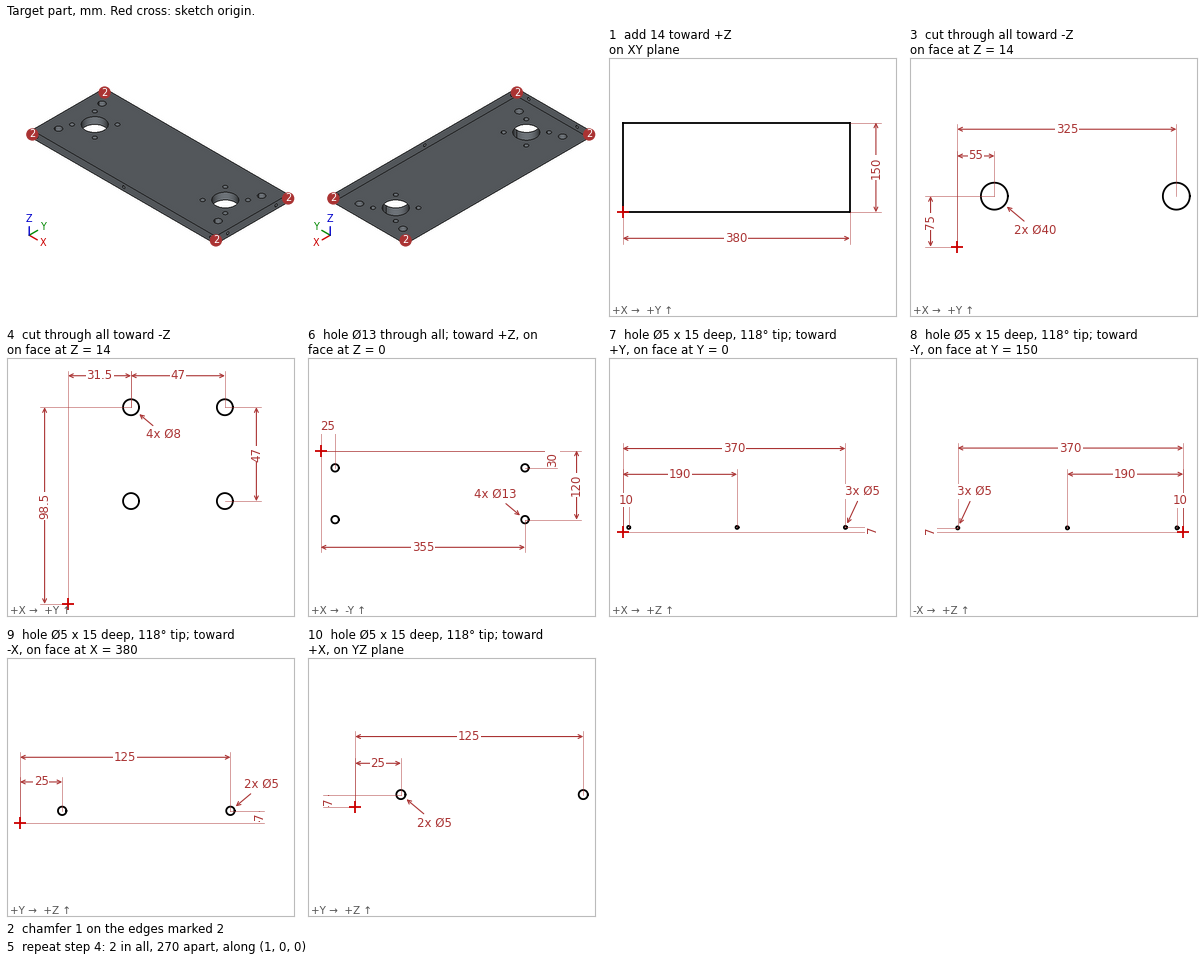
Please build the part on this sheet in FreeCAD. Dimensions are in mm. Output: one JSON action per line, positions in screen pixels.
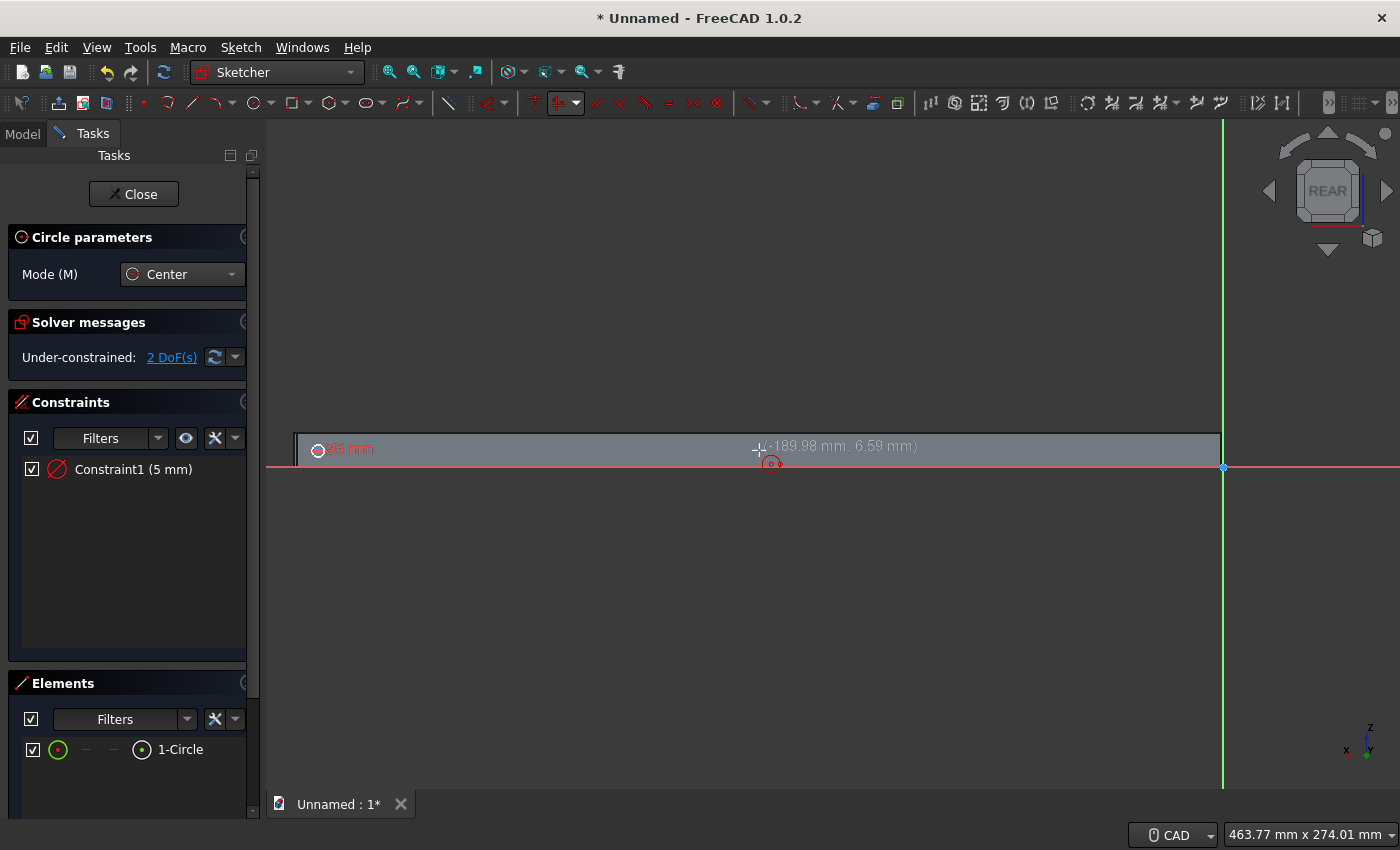
{"action": "left_click", "coordinate": [759, 450]}
{"action": "mouse_move", "coordinate": [763, 446]}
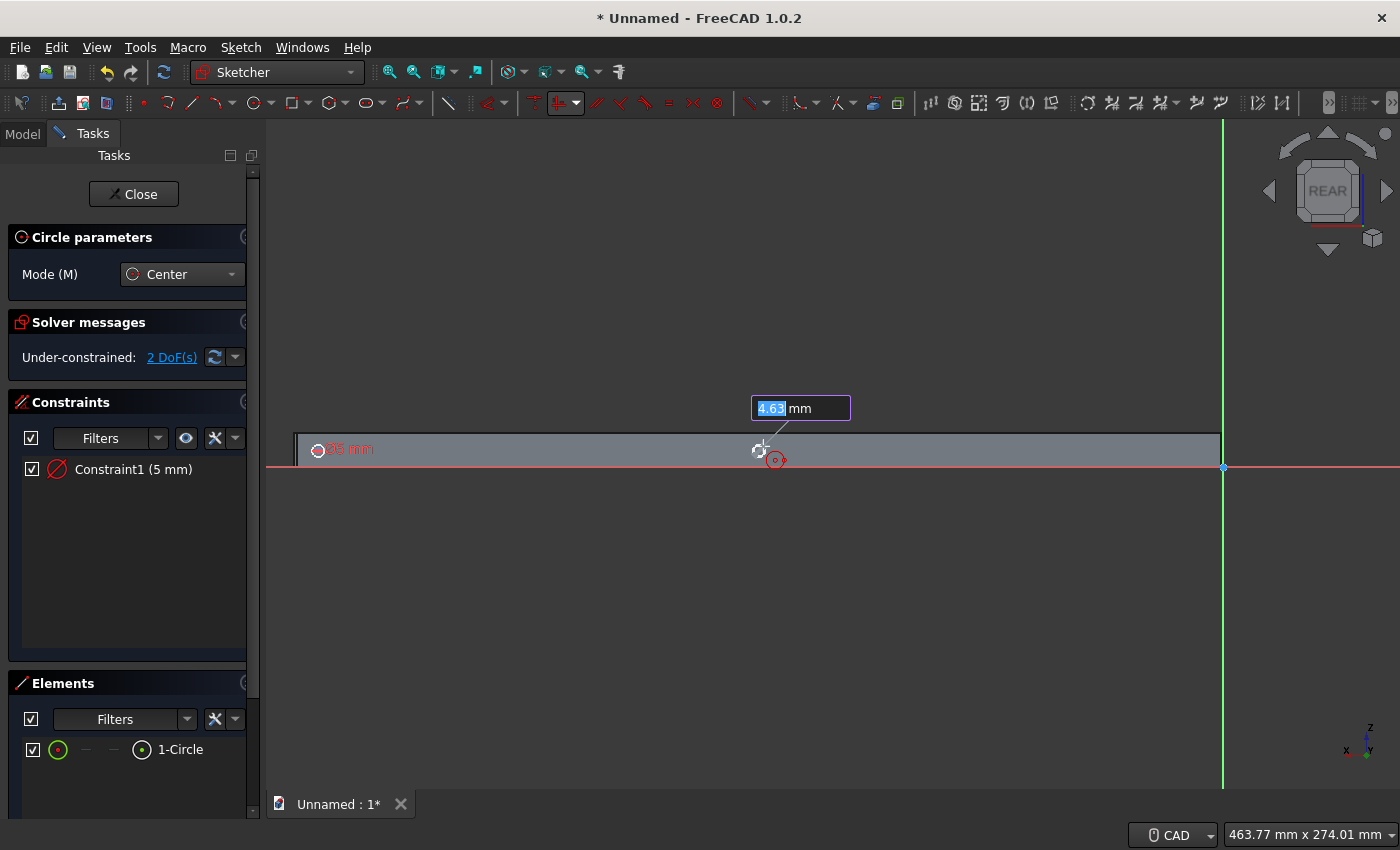
{"action": "type", "text": "5"}
{"action": "key", "text": "Return"}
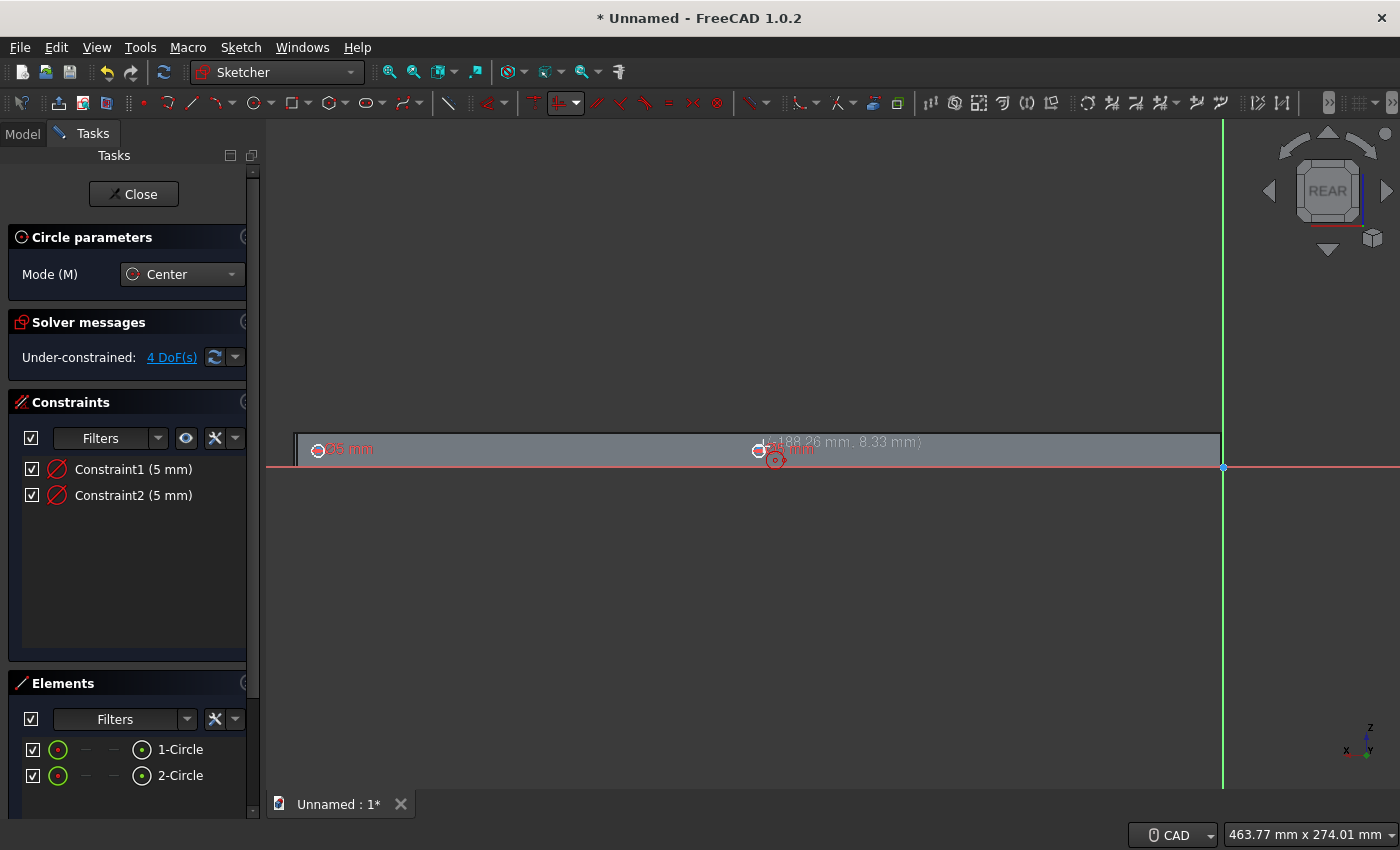
{"action": "scroll", "coordinate": [1199, 450], "scroll_direction": "up", "scroll_amount": 7}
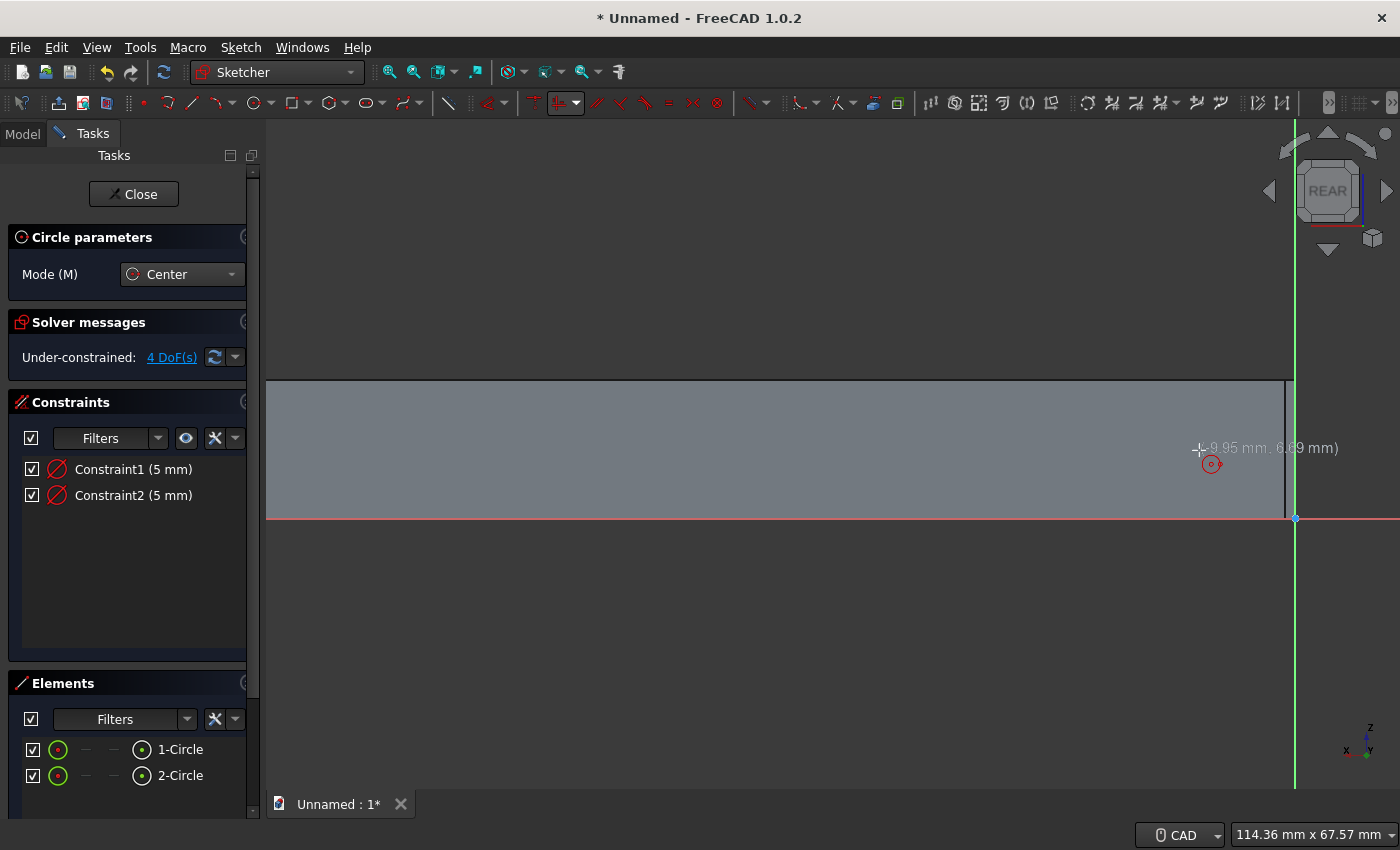
{"action": "scroll", "coordinate": [1025, 450], "scroll_direction": "down", "scroll_amount": 9}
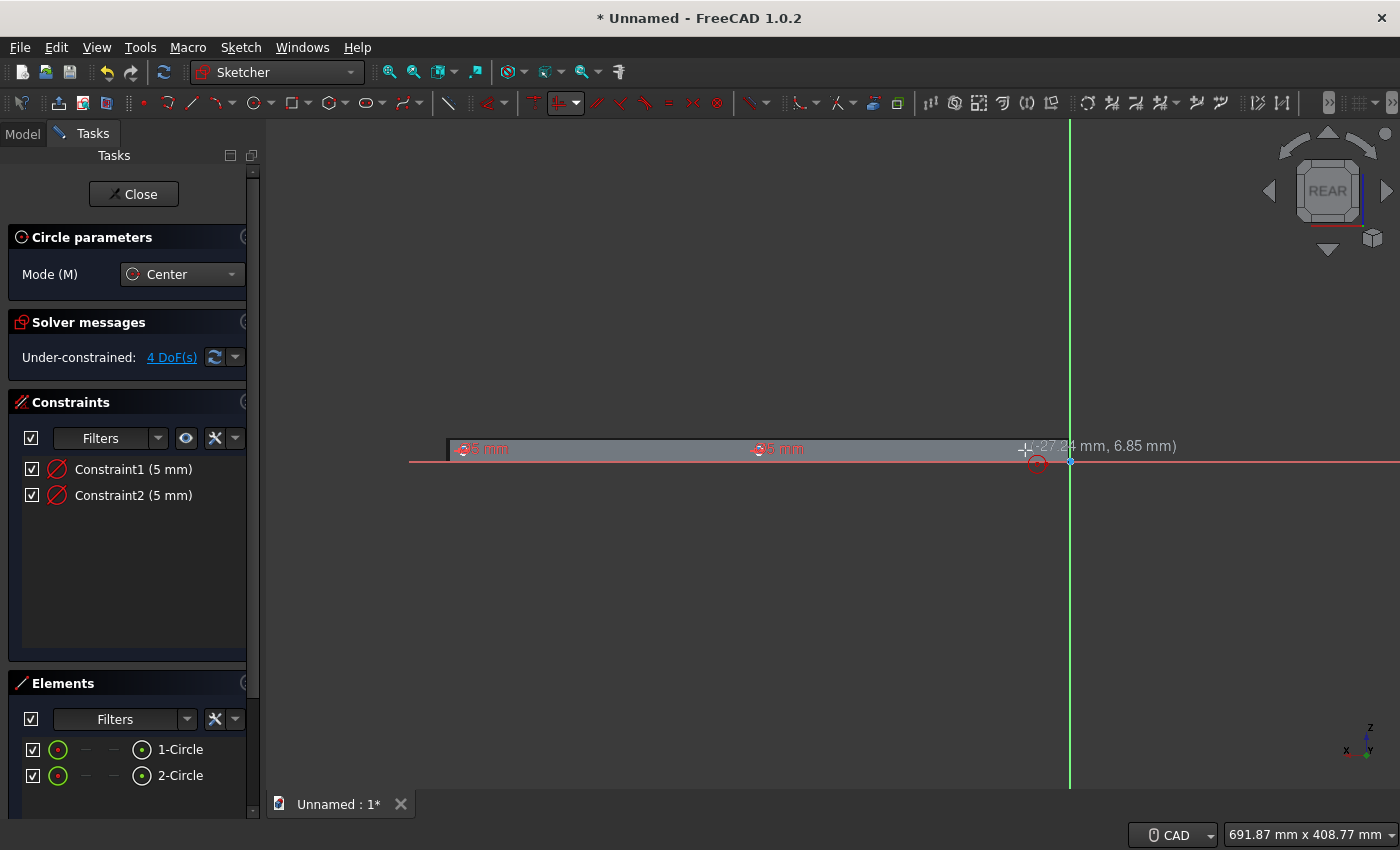
{"action": "scroll", "coordinate": [1054, 450], "scroll_direction": "up", "scroll_amount": 2}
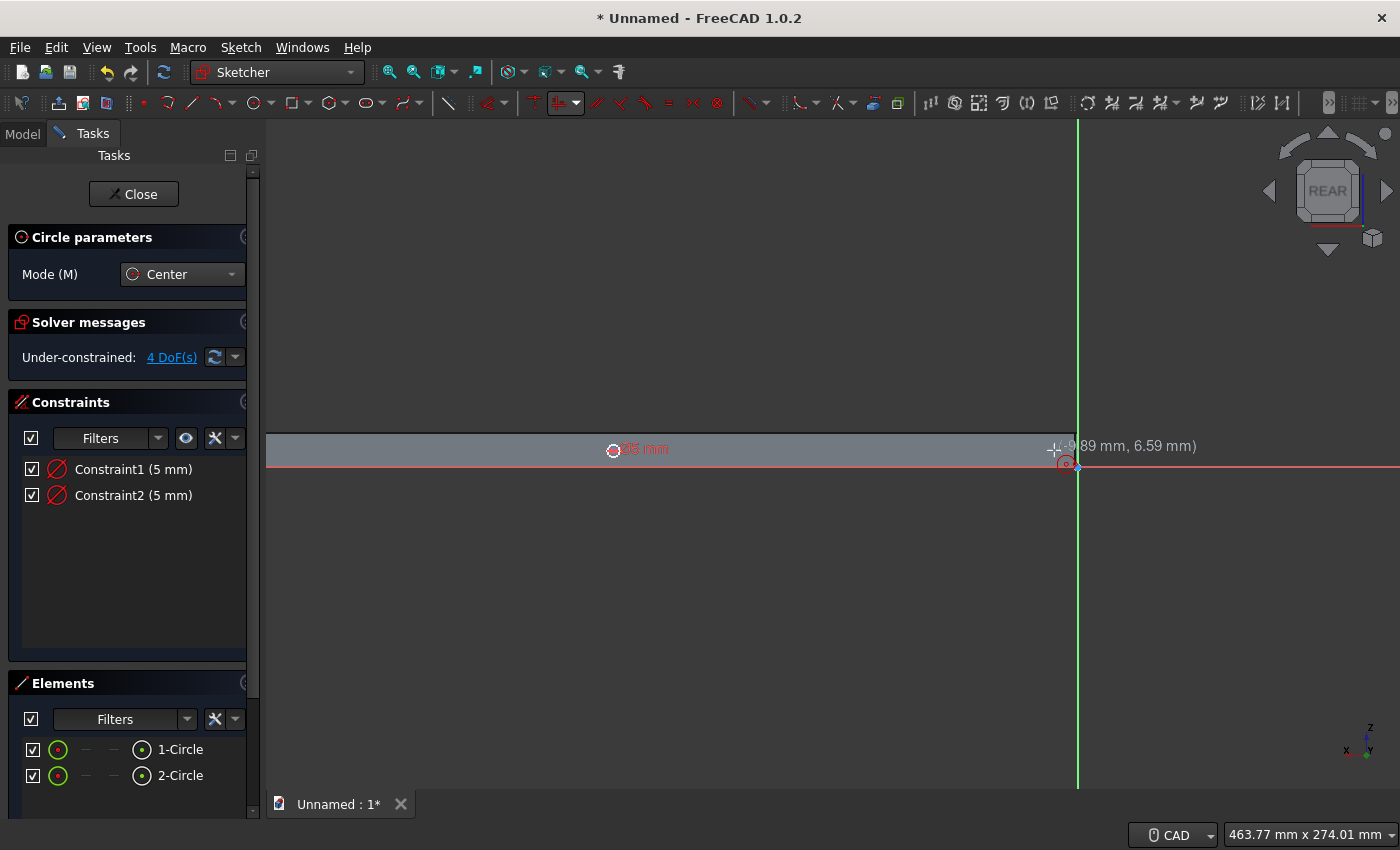
{"action": "left_click", "coordinate": [1053, 450]}
{"action": "mouse_move", "coordinate": [1058, 446]}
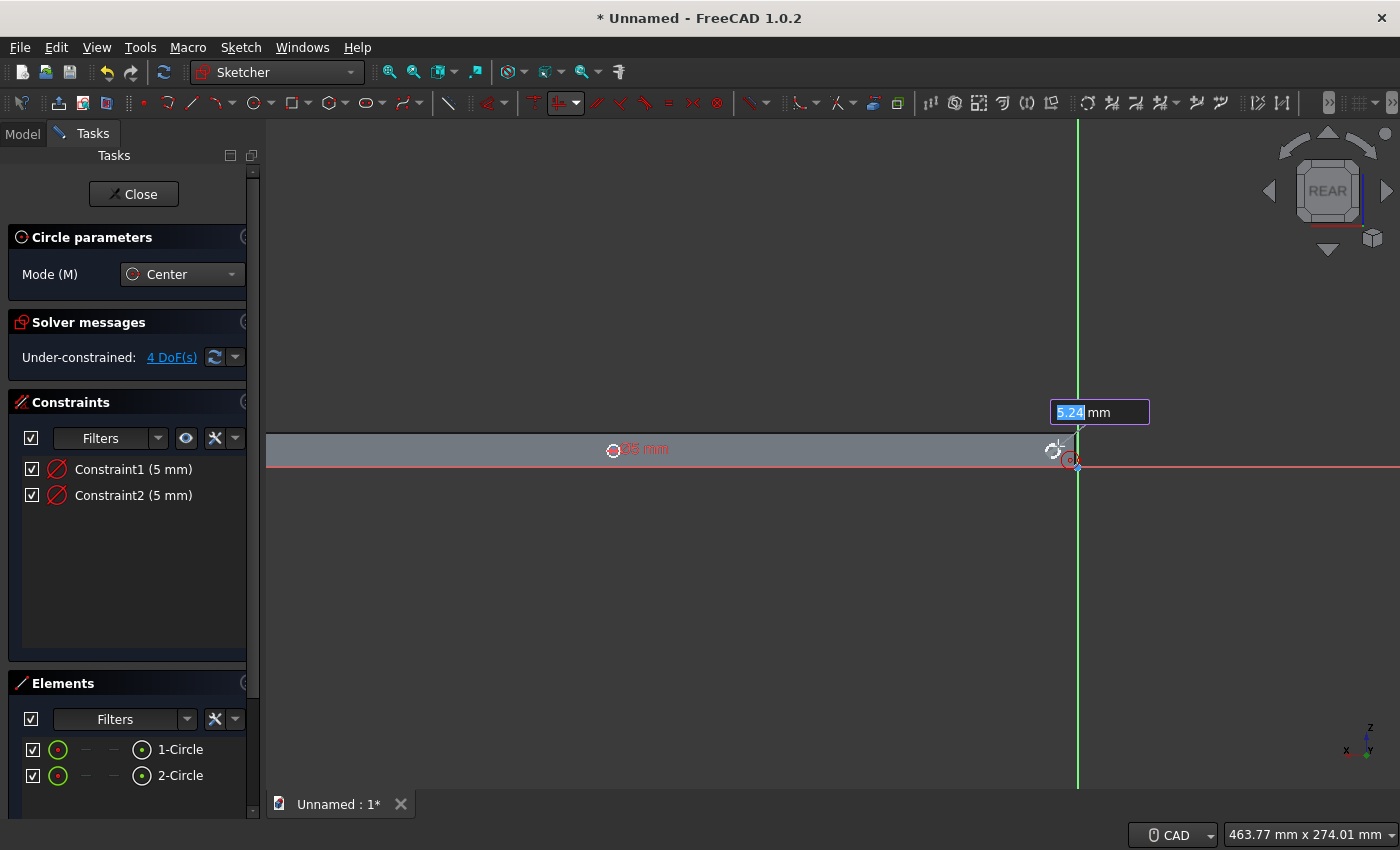
{"action": "type", "text": "5"}
{"action": "key", "text": "Return"}
{"action": "key", "text": "Escape"}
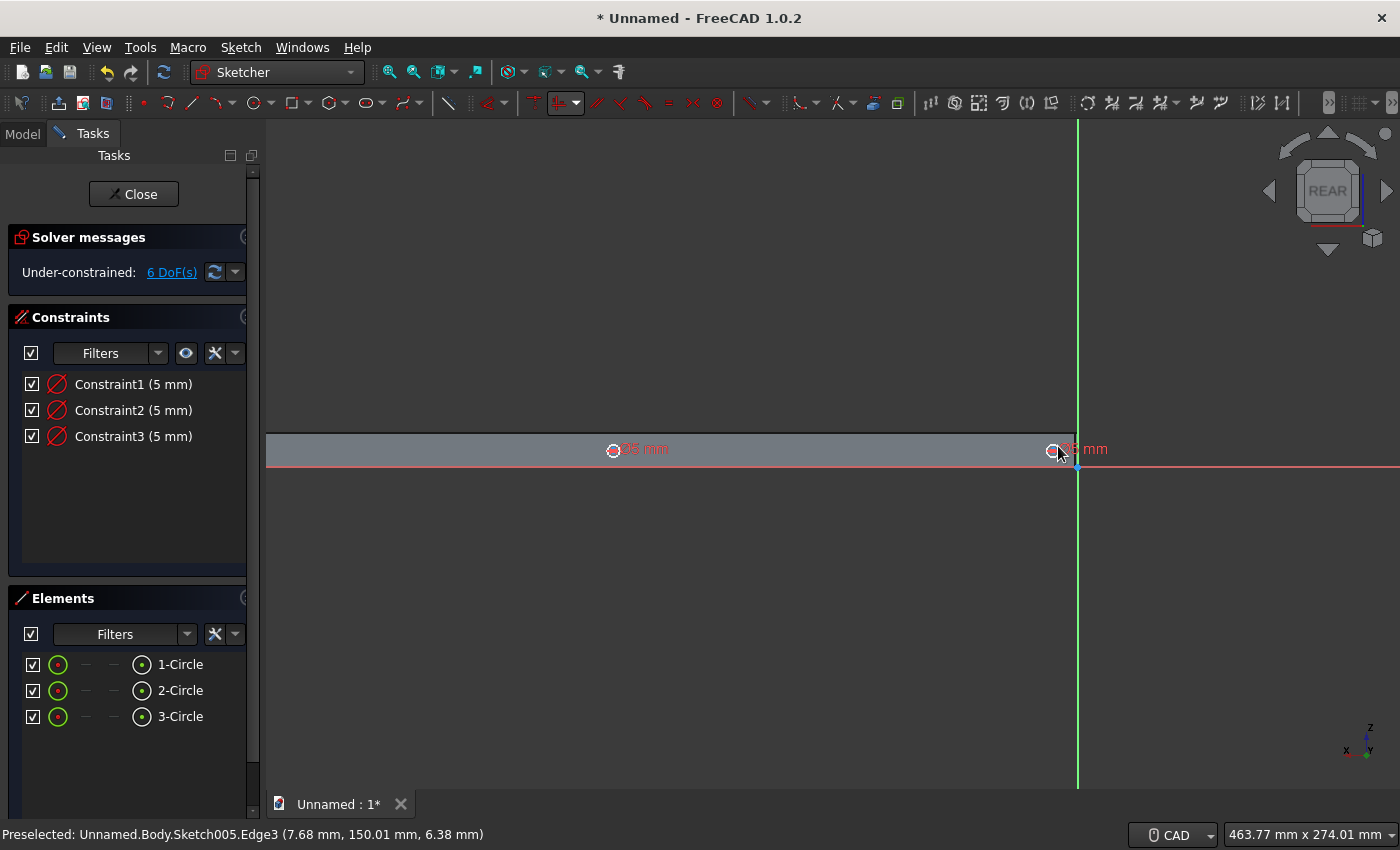
{"action": "scroll", "coordinate": [1053, 450], "scroll_direction": "down", "scroll_amount": 2}